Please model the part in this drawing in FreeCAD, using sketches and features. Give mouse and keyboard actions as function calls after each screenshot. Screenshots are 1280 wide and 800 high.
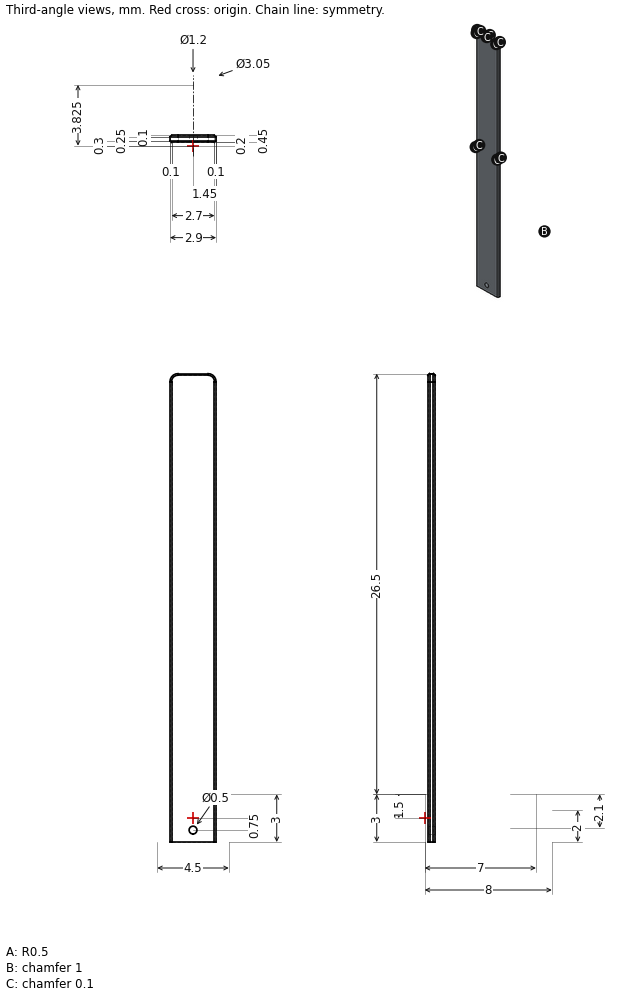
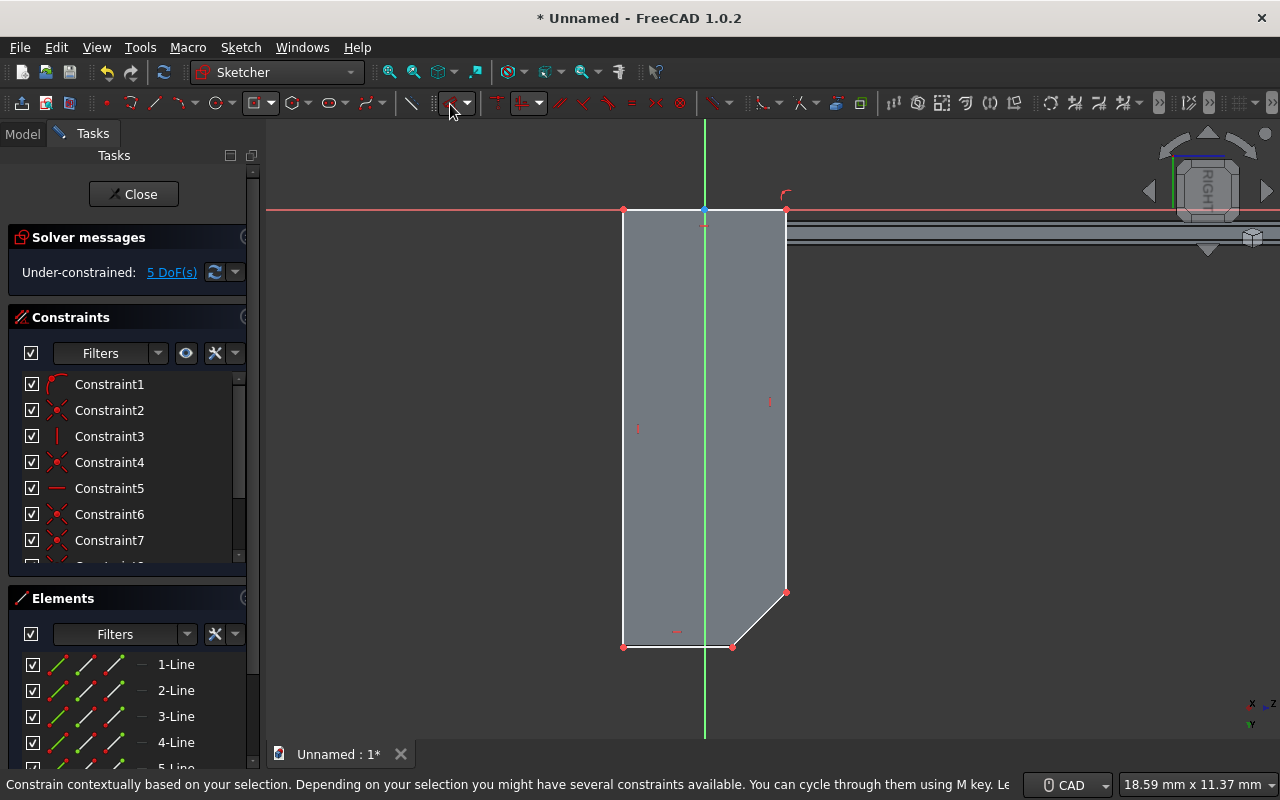
click(737, 210)
click(667, 176)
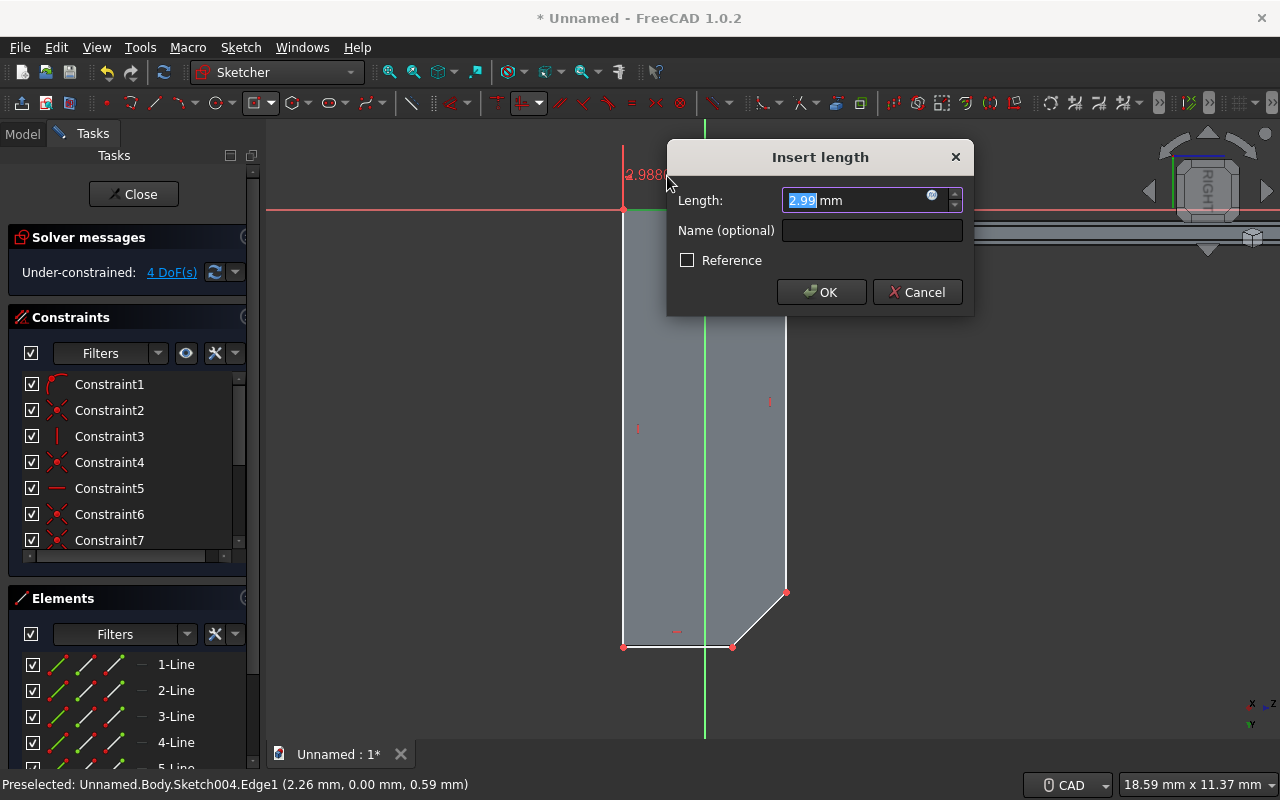
text(3)
key(Return)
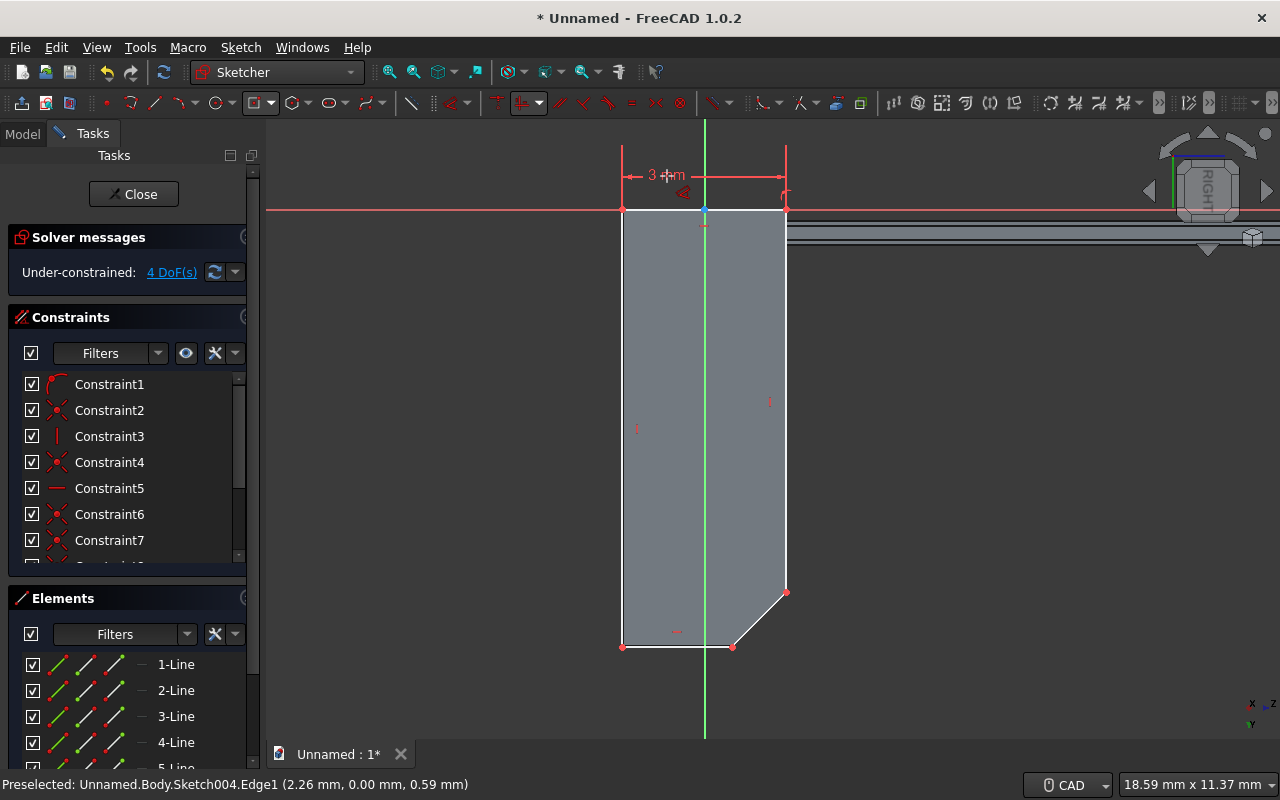
click(622, 341)
click(588, 428)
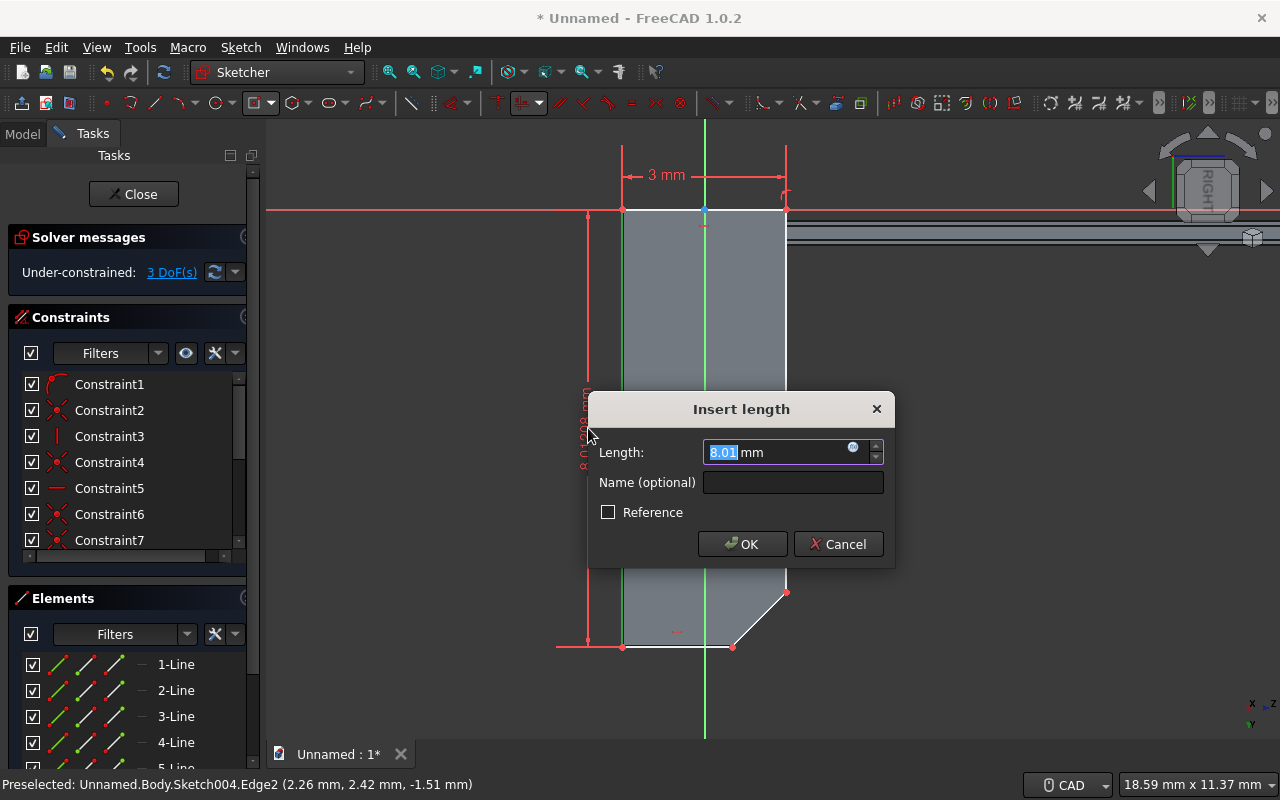
text(8)
key(Return)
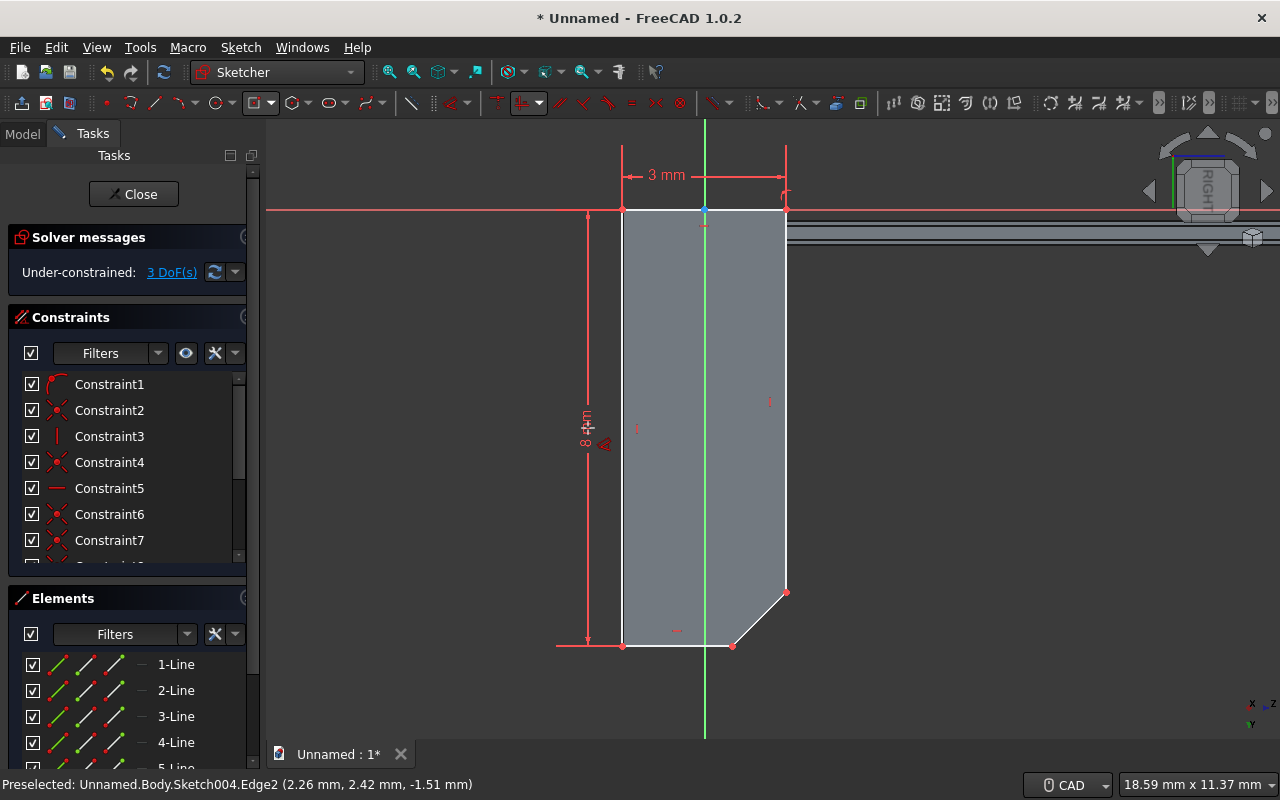
click(655, 646)
click(677, 680)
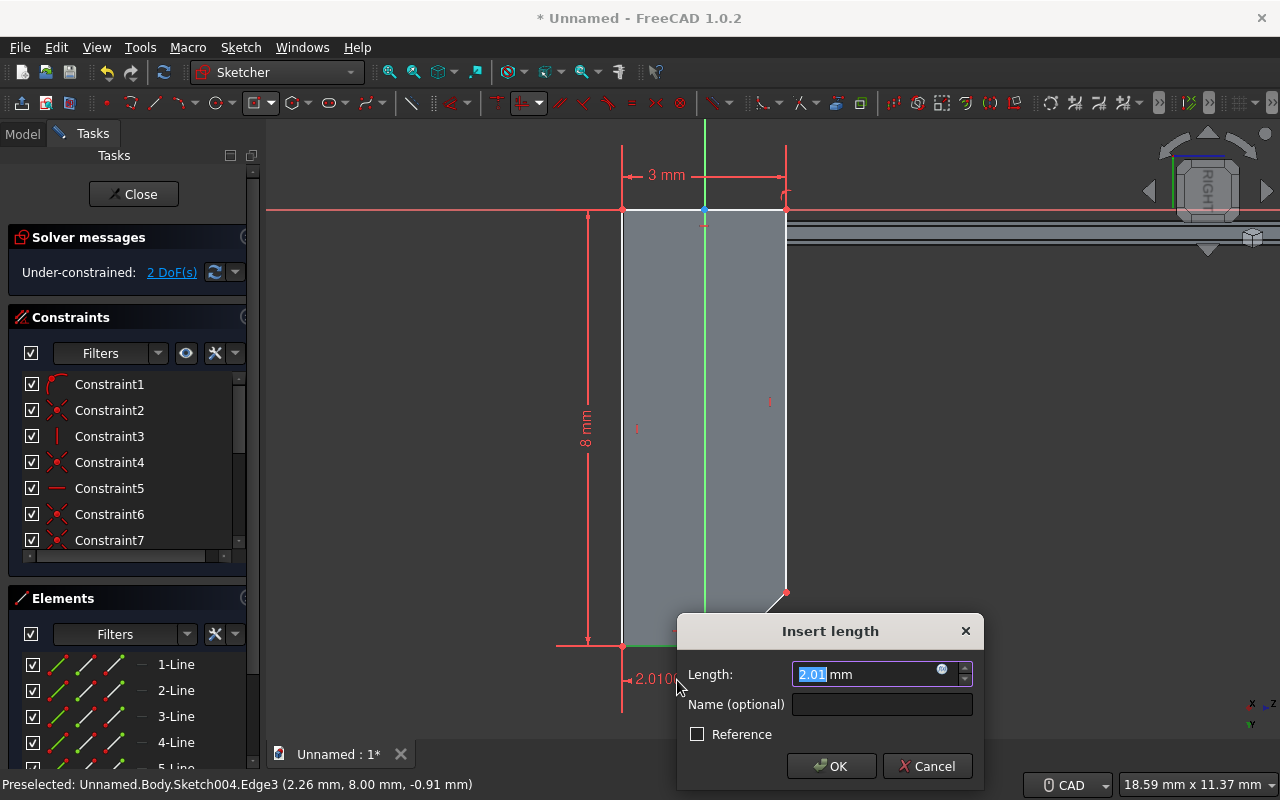
text(2)
key(Return)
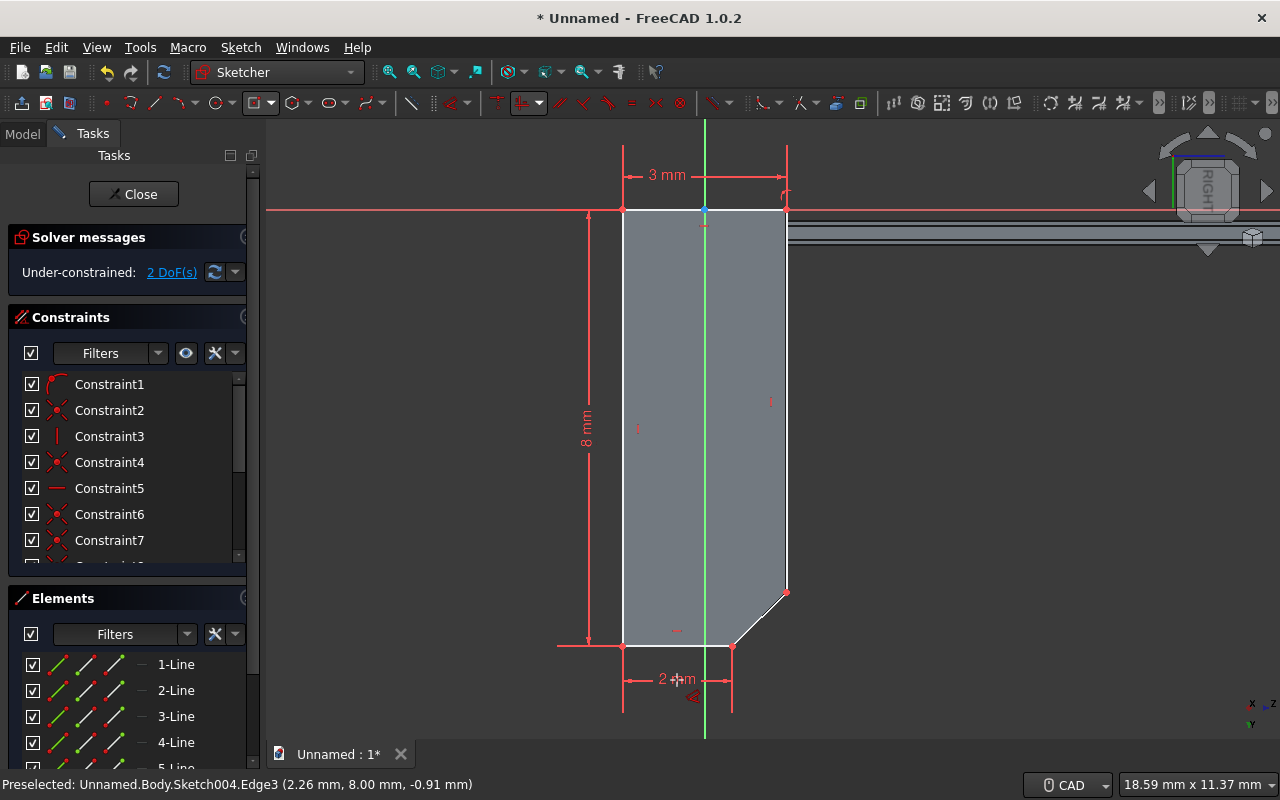
click(787, 478)
click(821, 401)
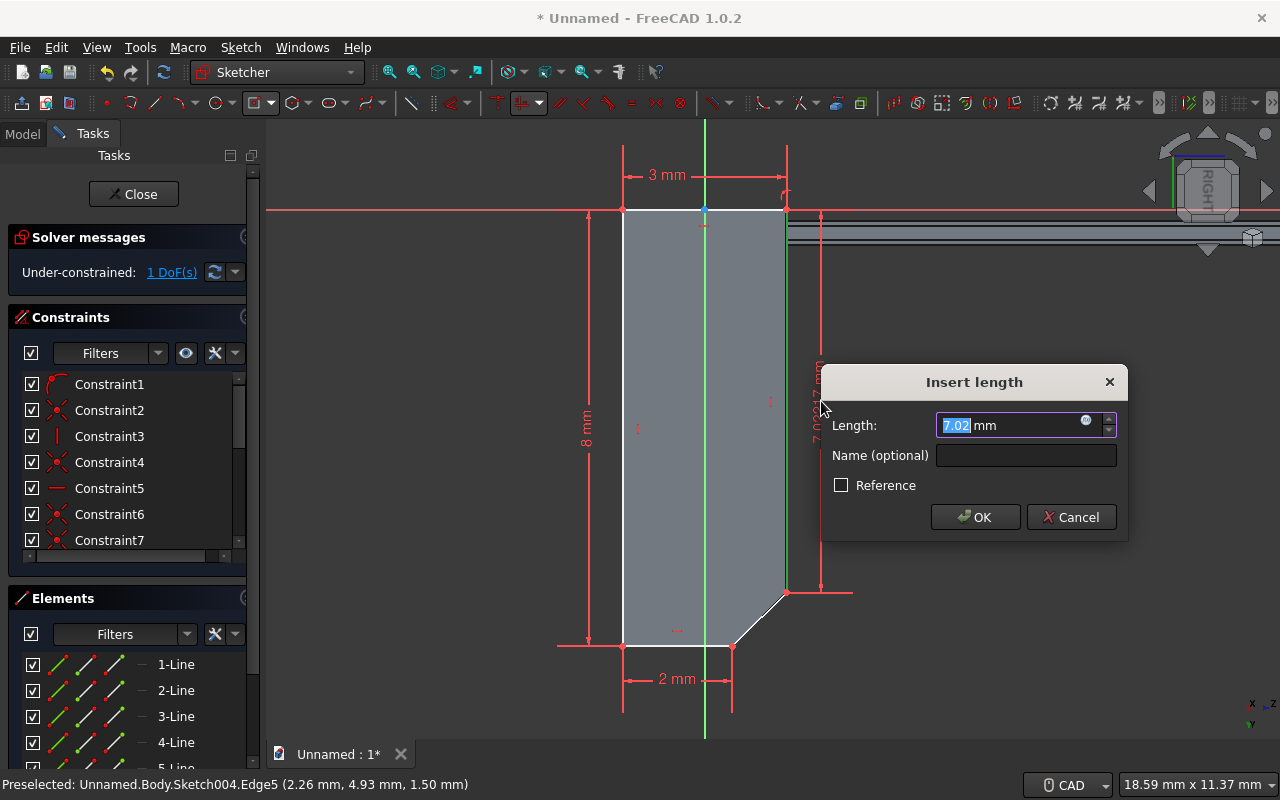
text(7)
key(Return)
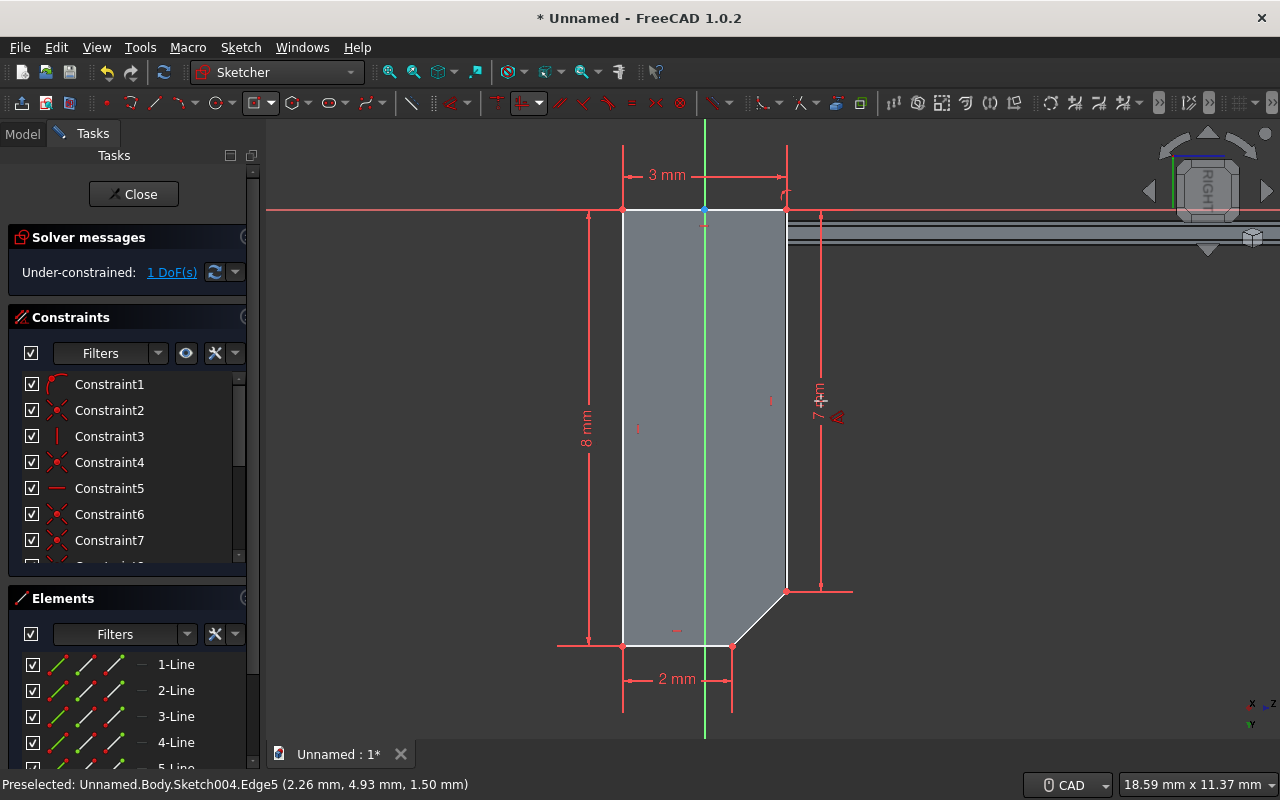
click(787, 210)
click(746, 176)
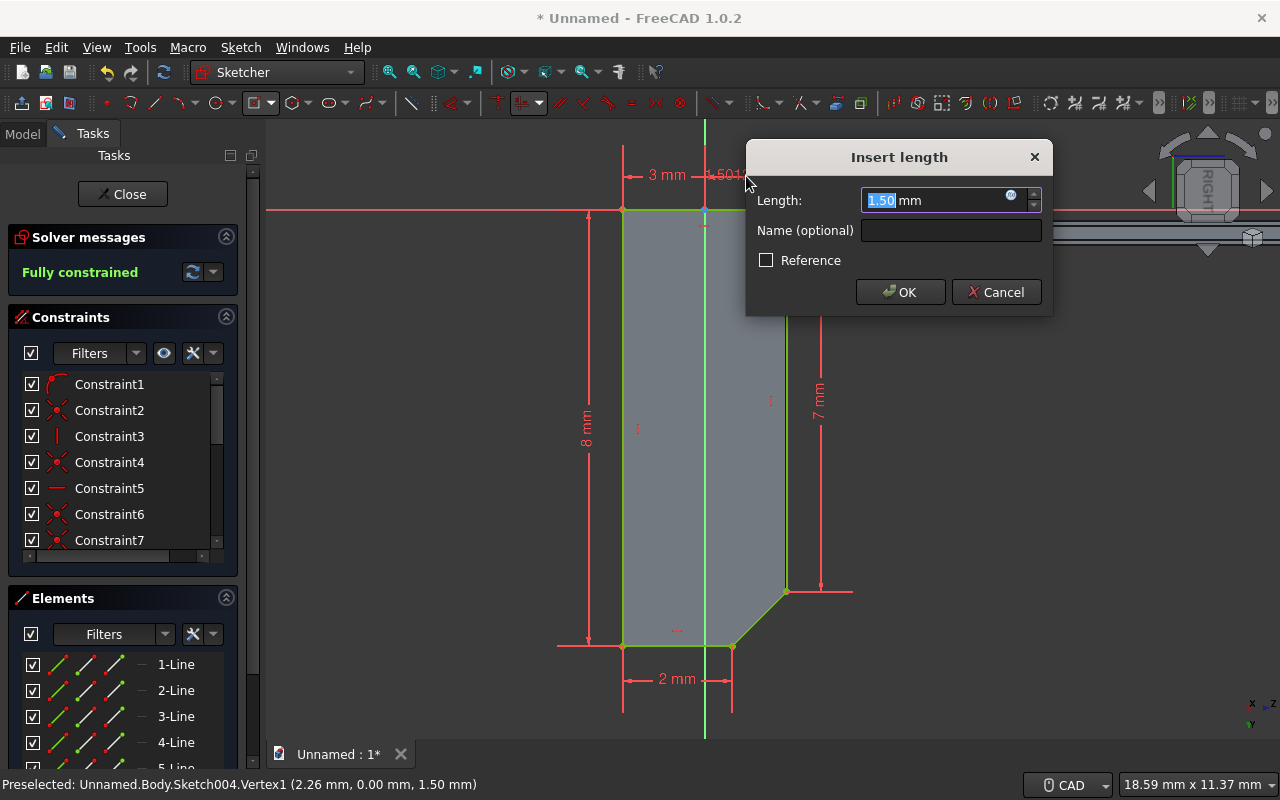
text(1.5)
key(Return)
key(Escape)